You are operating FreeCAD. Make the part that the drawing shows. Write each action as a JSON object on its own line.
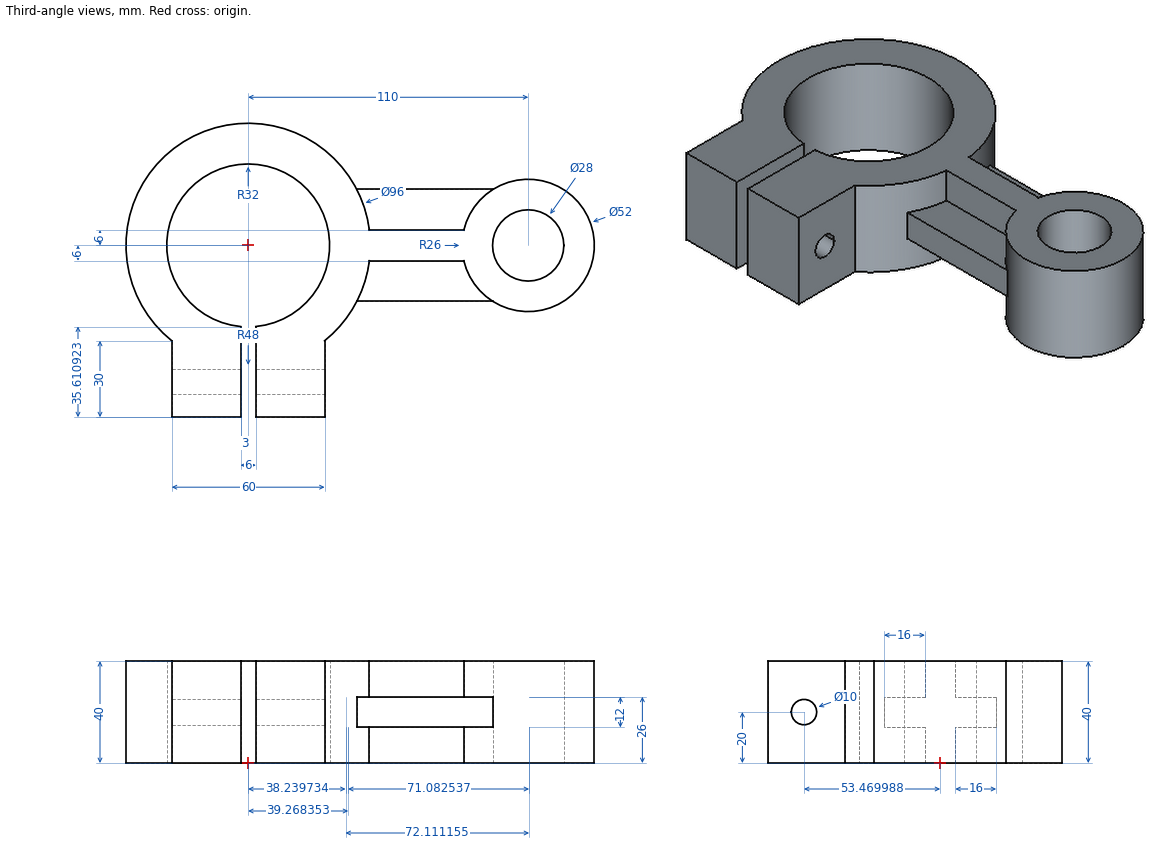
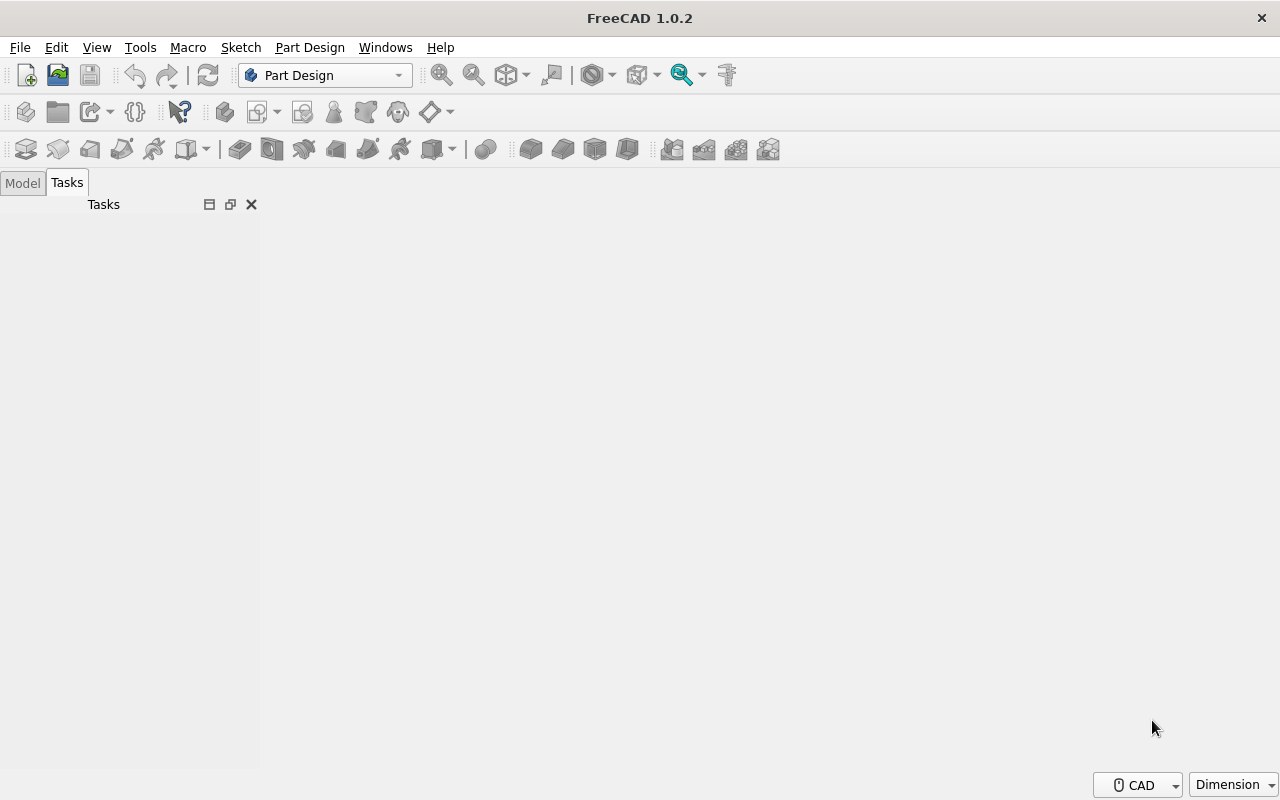
{"action": "left_click", "coordinate": [26, 76]}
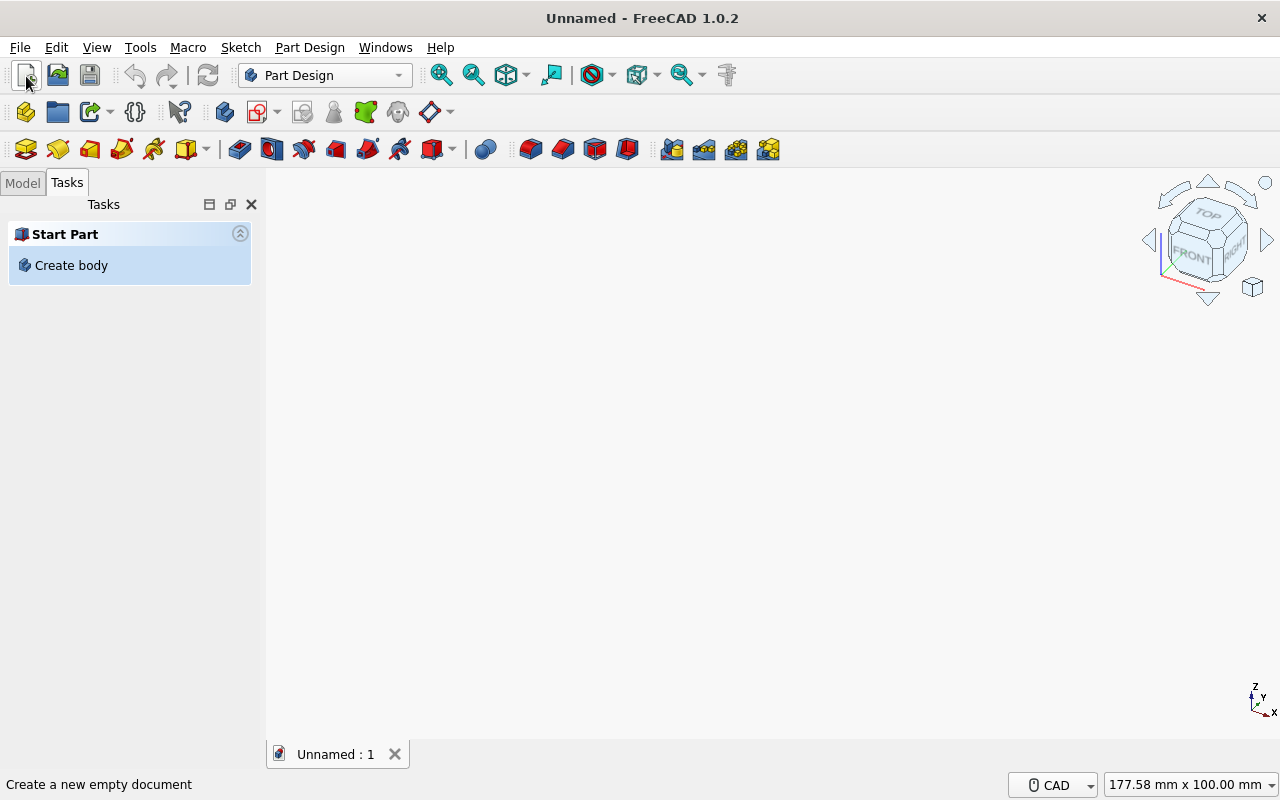
{"action": "left_click", "coordinate": [258, 112]}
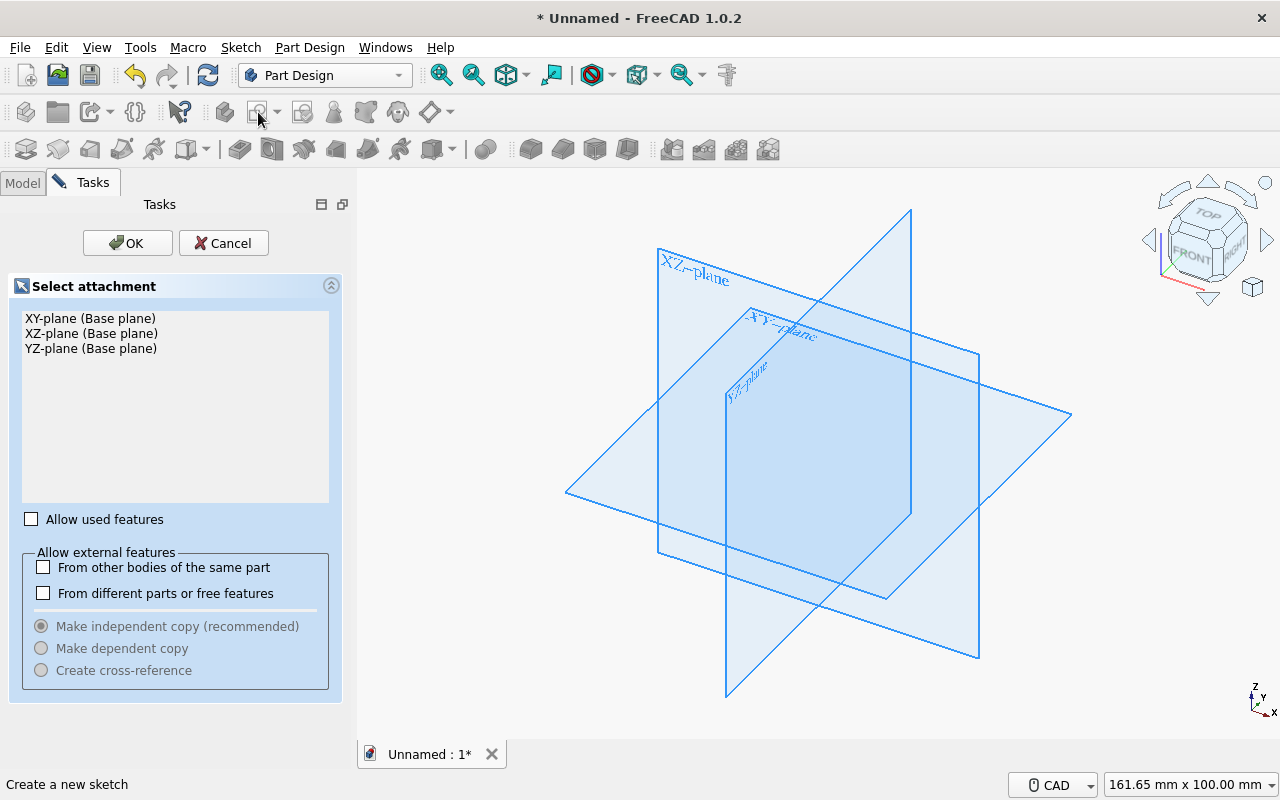
{"action": "left_click", "coordinate": [82, 318]}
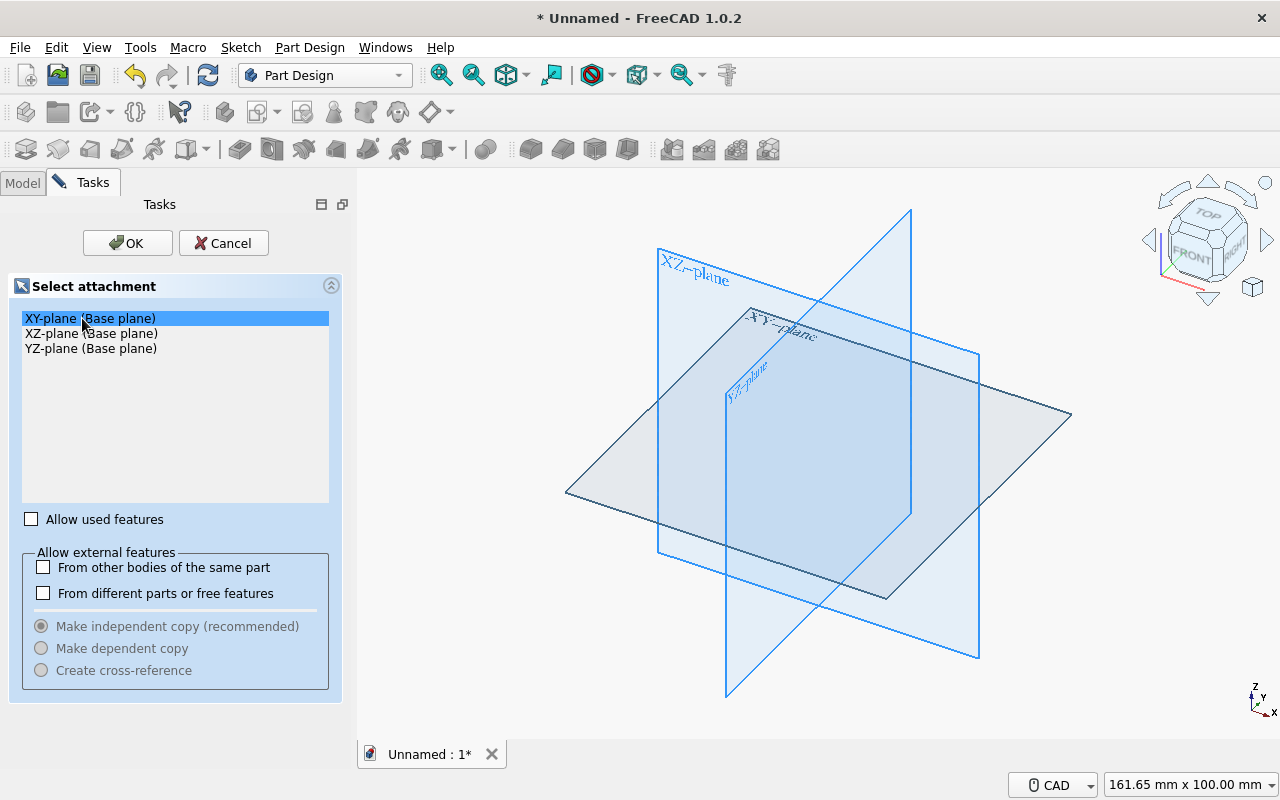
{"action": "left_click", "coordinate": [128, 243]}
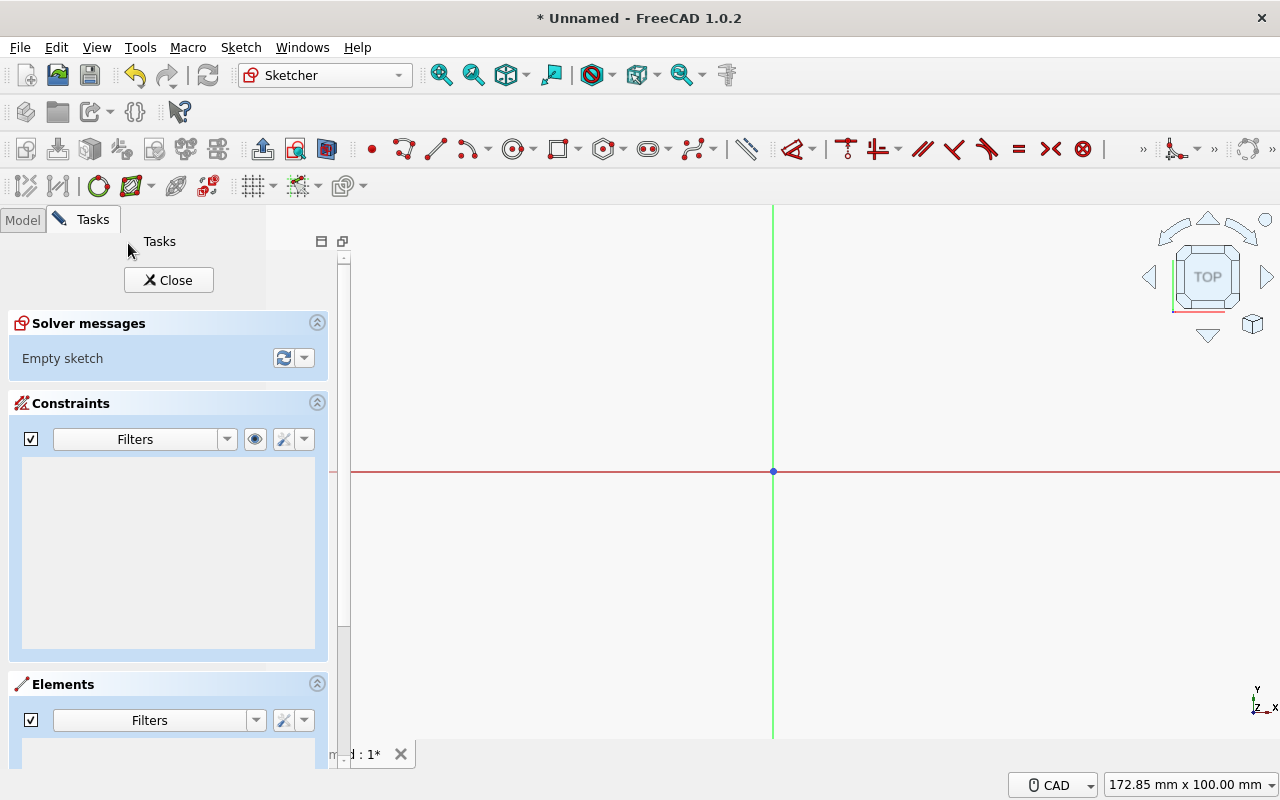
{"action": "scroll", "coordinate": [565, 472], "scroll_direction": "down", "scroll_amount": 2}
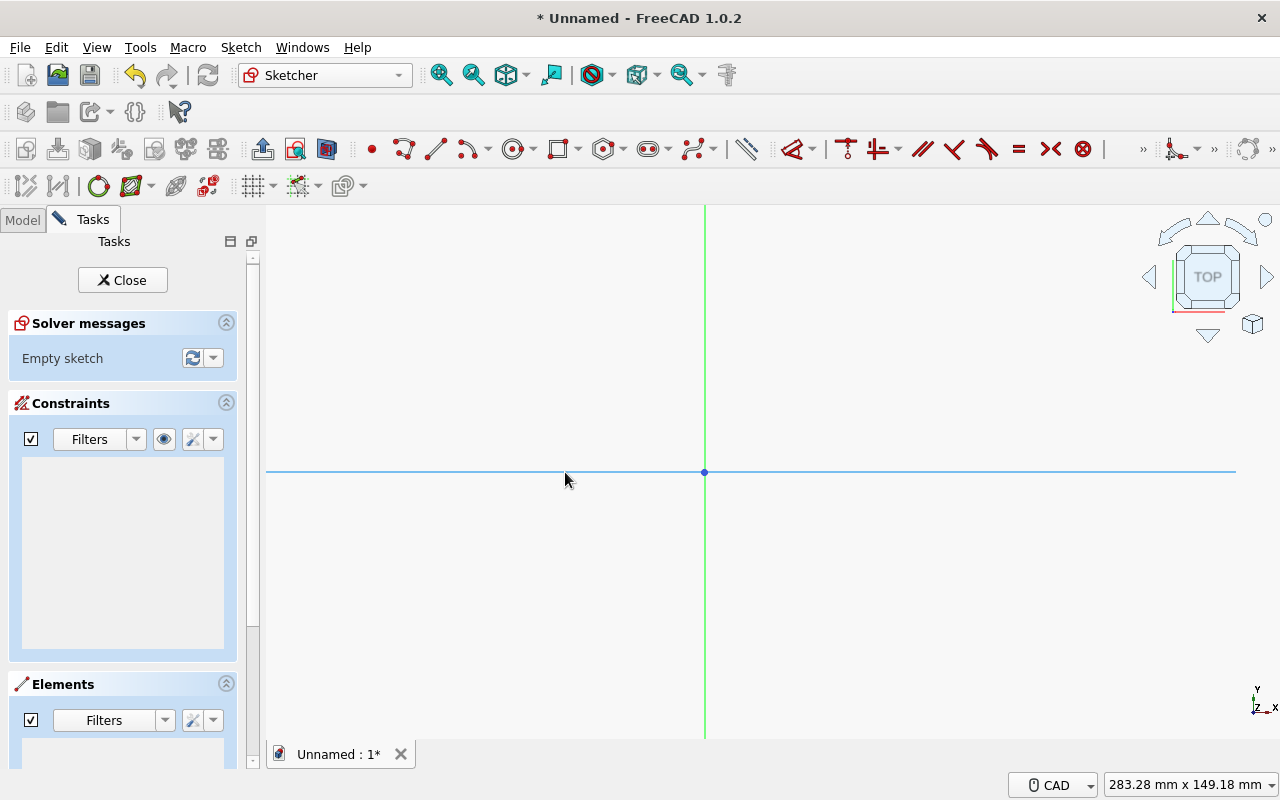
{"action": "left_click", "coordinate": [514, 150]}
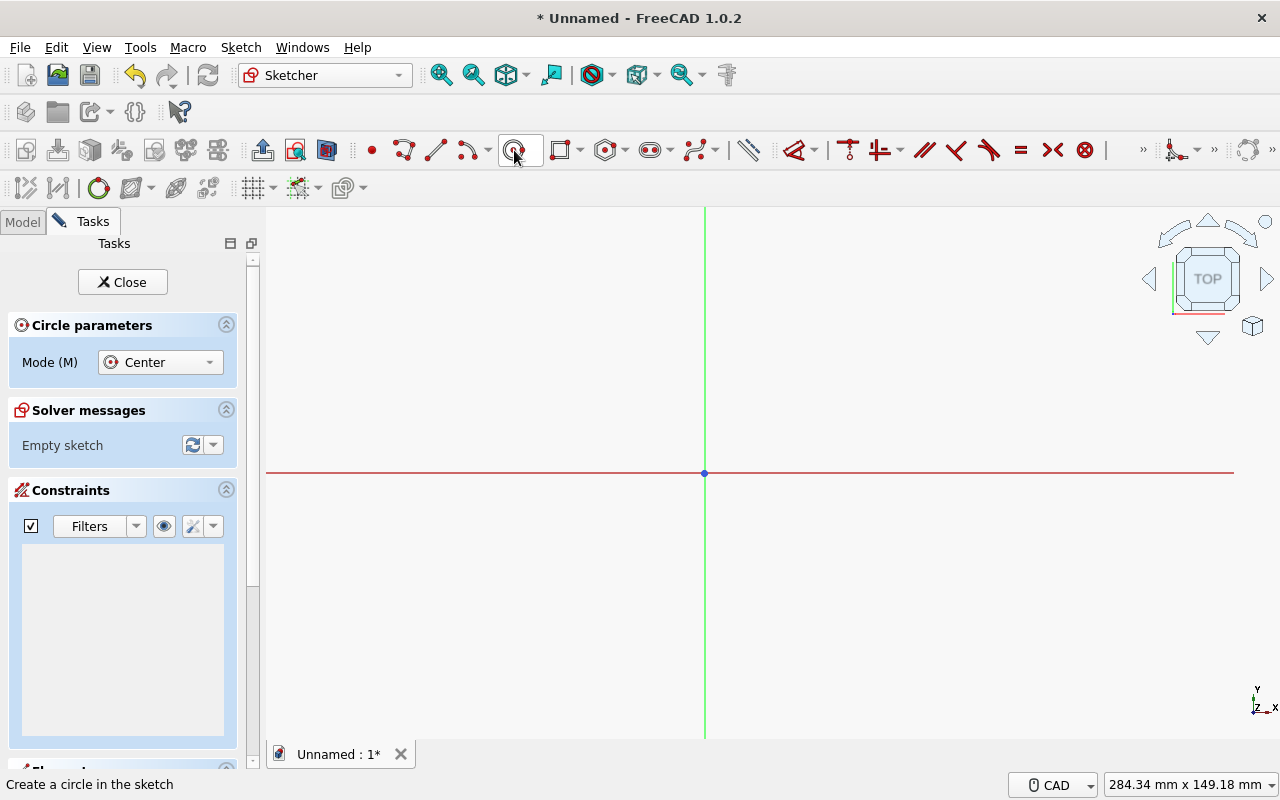
{"action": "left_click", "coordinate": [705, 473]}
{"action": "left_click", "coordinate": [826, 352]}
{"action": "key", "text": "Escape"}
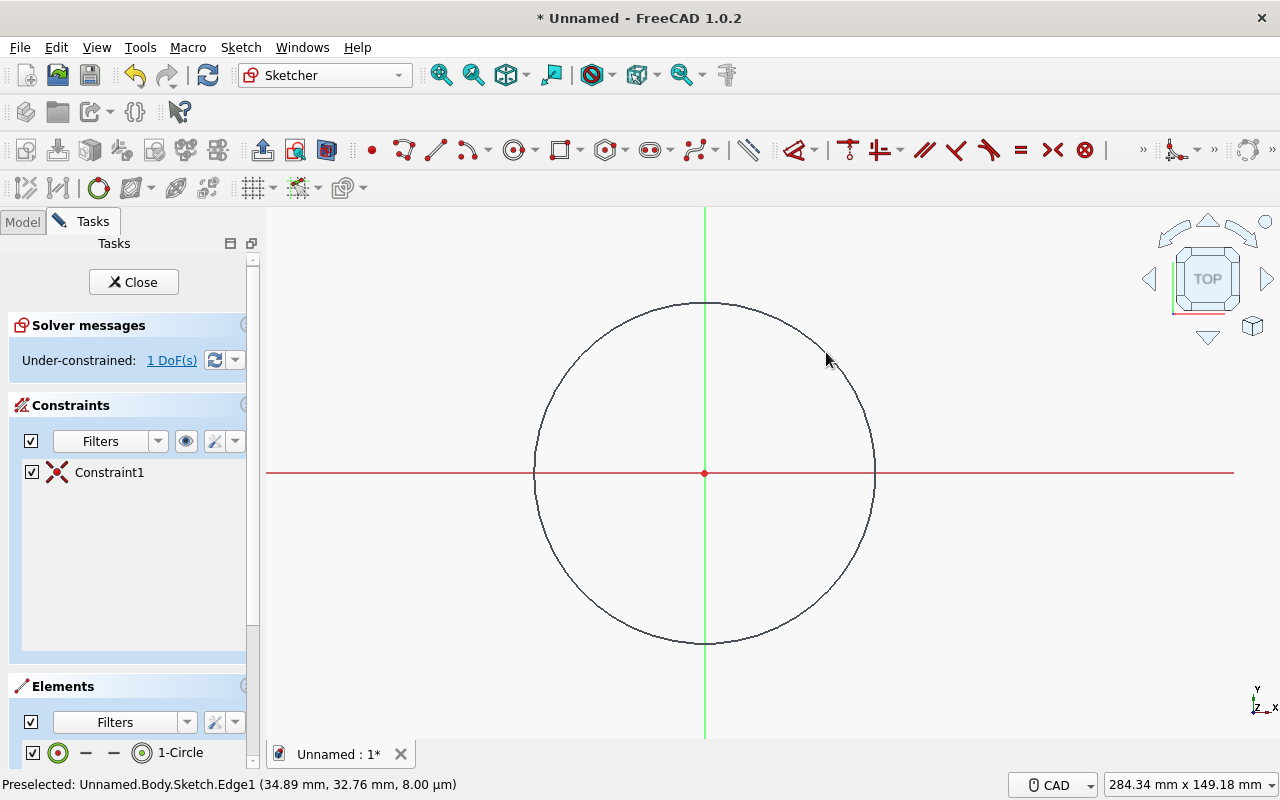
{"action": "left_click", "coordinate": [794, 150]}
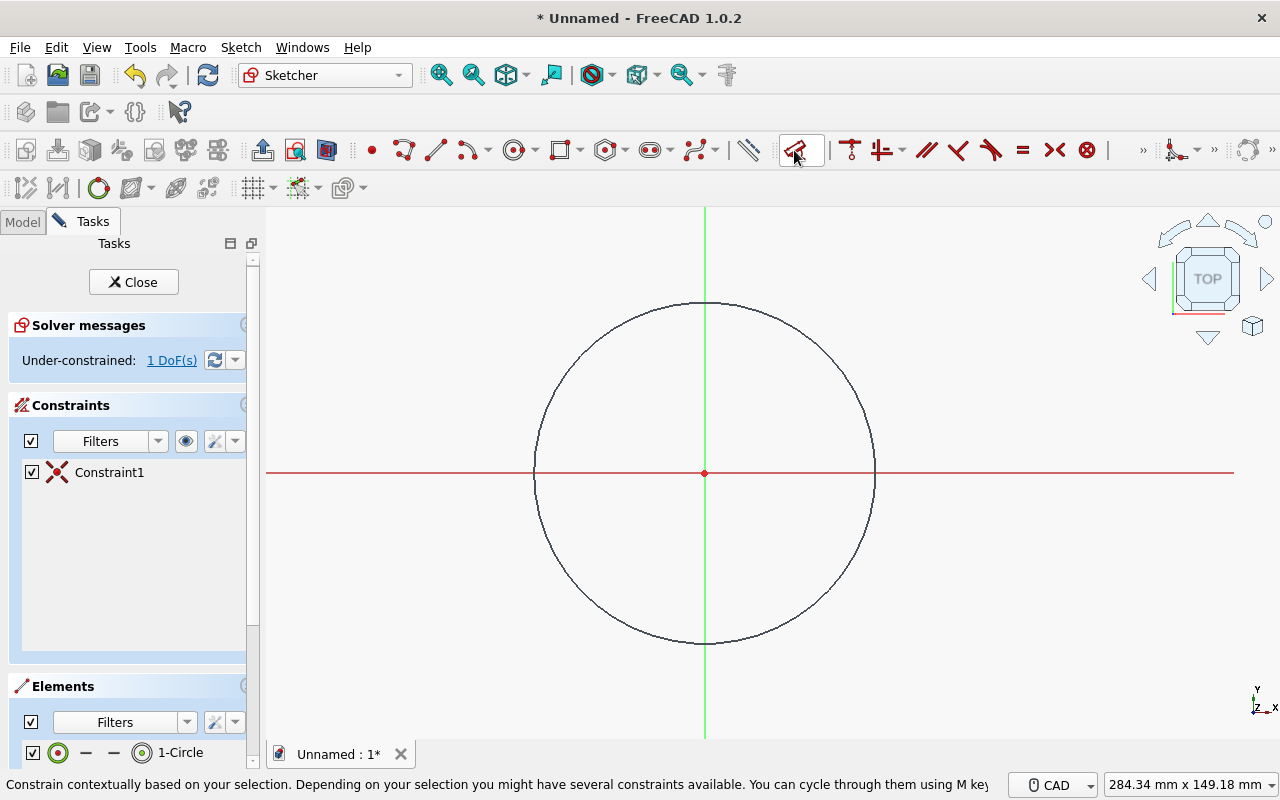
{"action": "left_click", "coordinate": [825, 352]}
{"action": "left_click", "coordinate": [848, 329]}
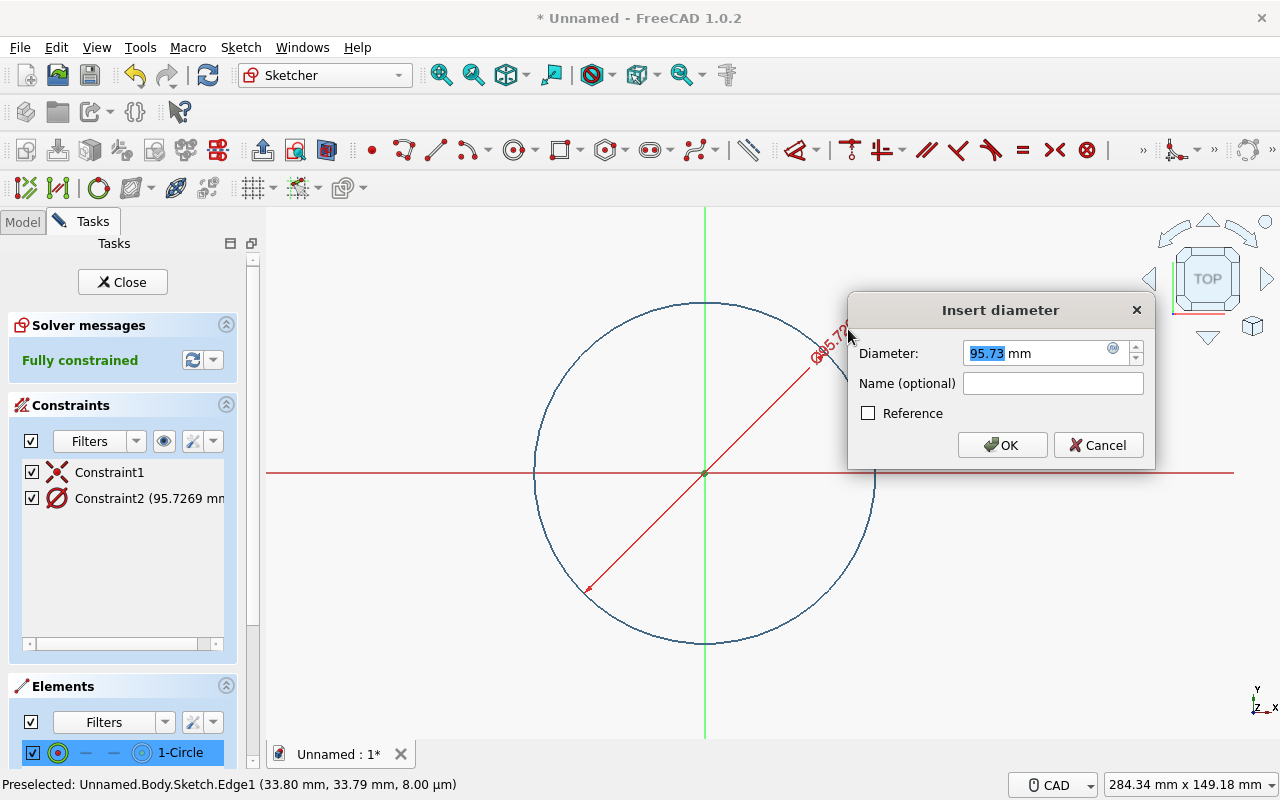
{"action": "type", "text": "96"}
{"action": "key", "text": "Return"}
{"action": "key", "text": "Escape"}